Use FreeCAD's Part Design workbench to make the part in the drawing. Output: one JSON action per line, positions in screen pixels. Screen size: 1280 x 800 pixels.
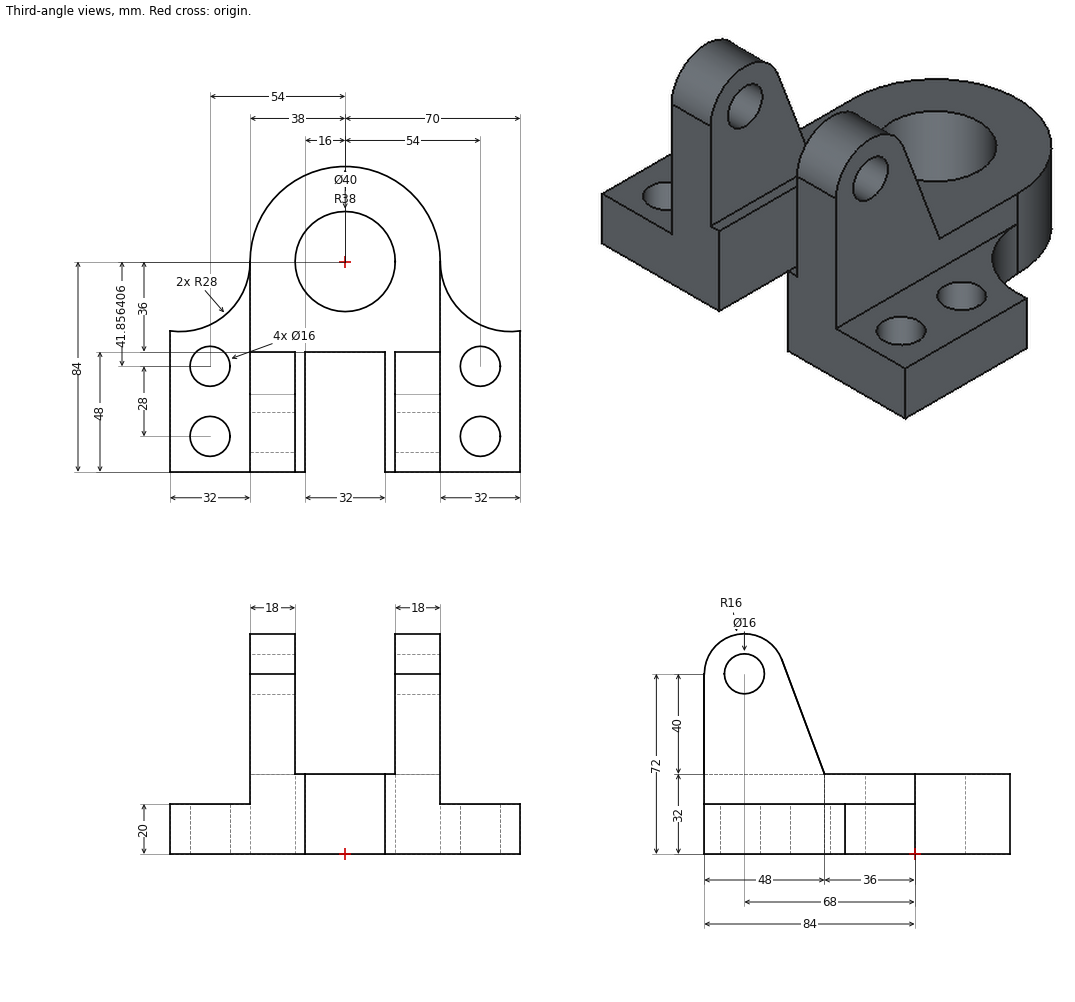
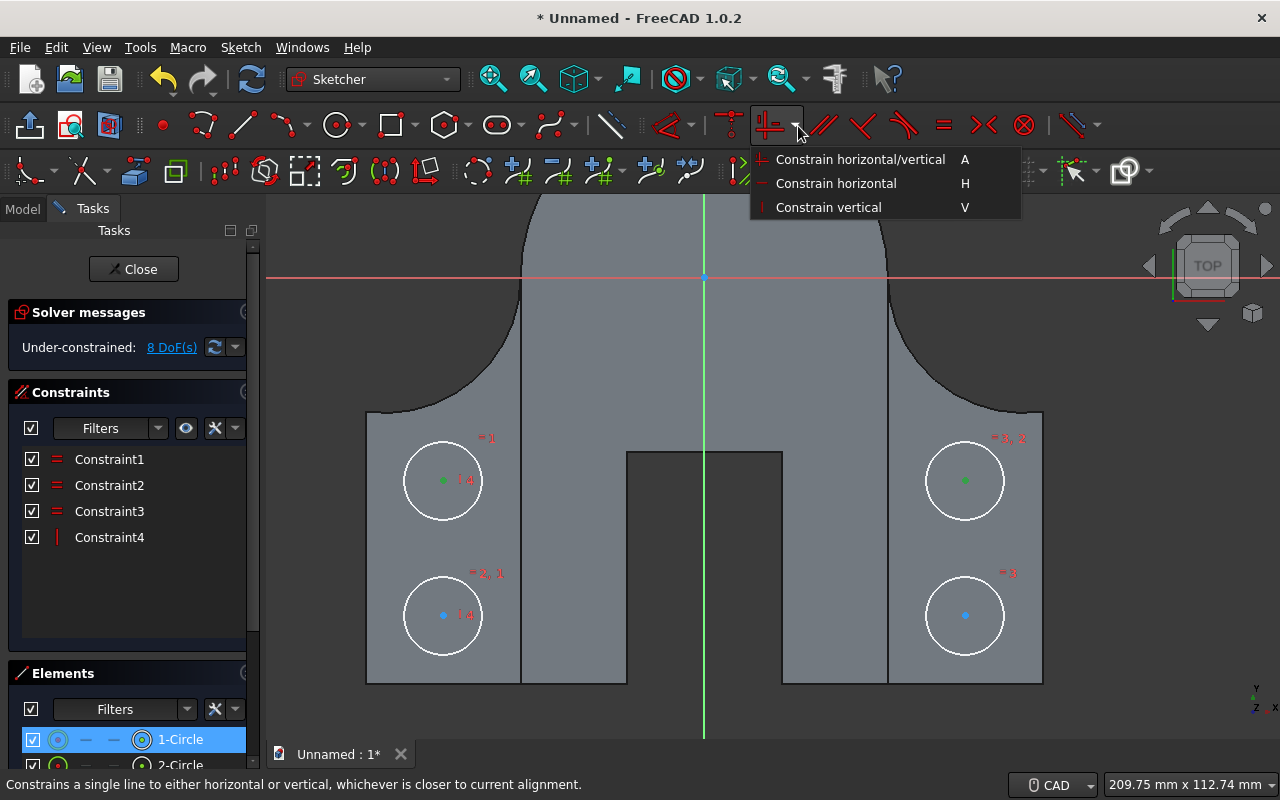
{"action": "left_click", "coordinate": [886, 183]}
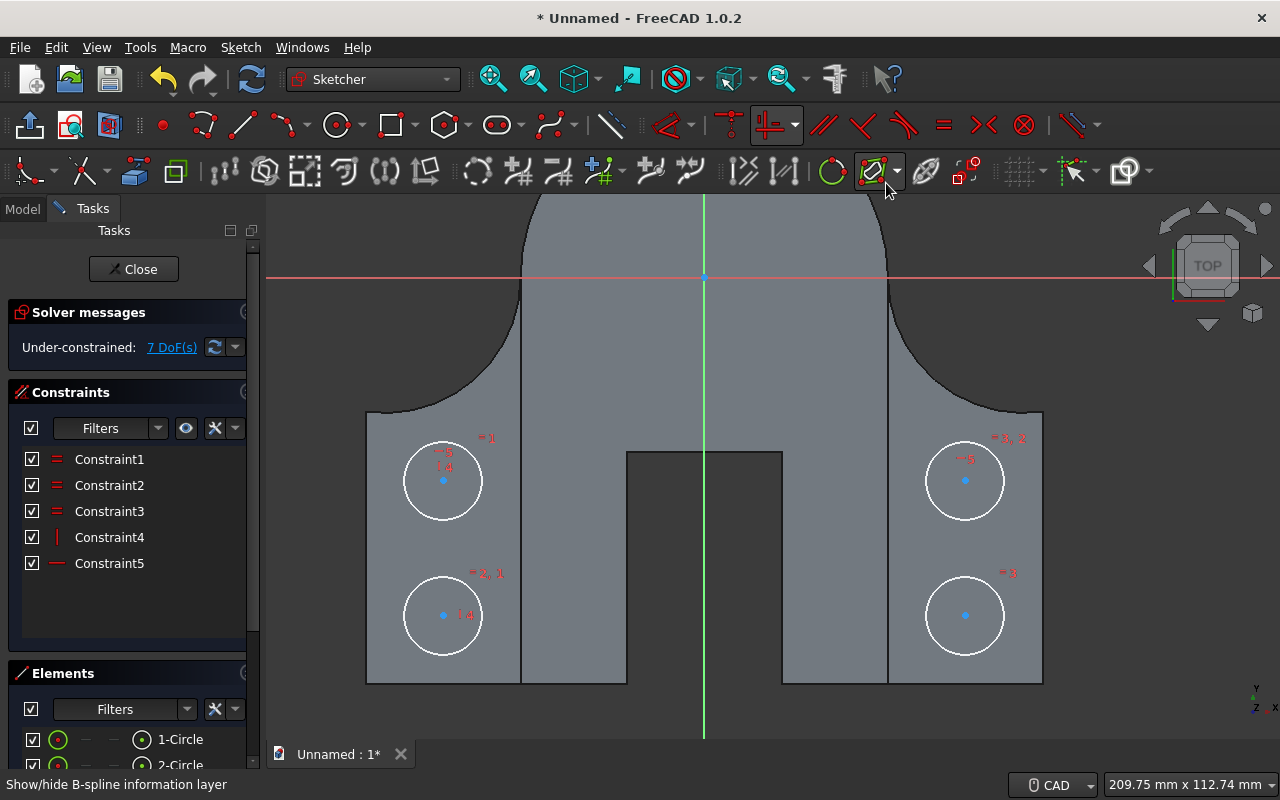
{"action": "left_click", "coordinate": [965, 481]}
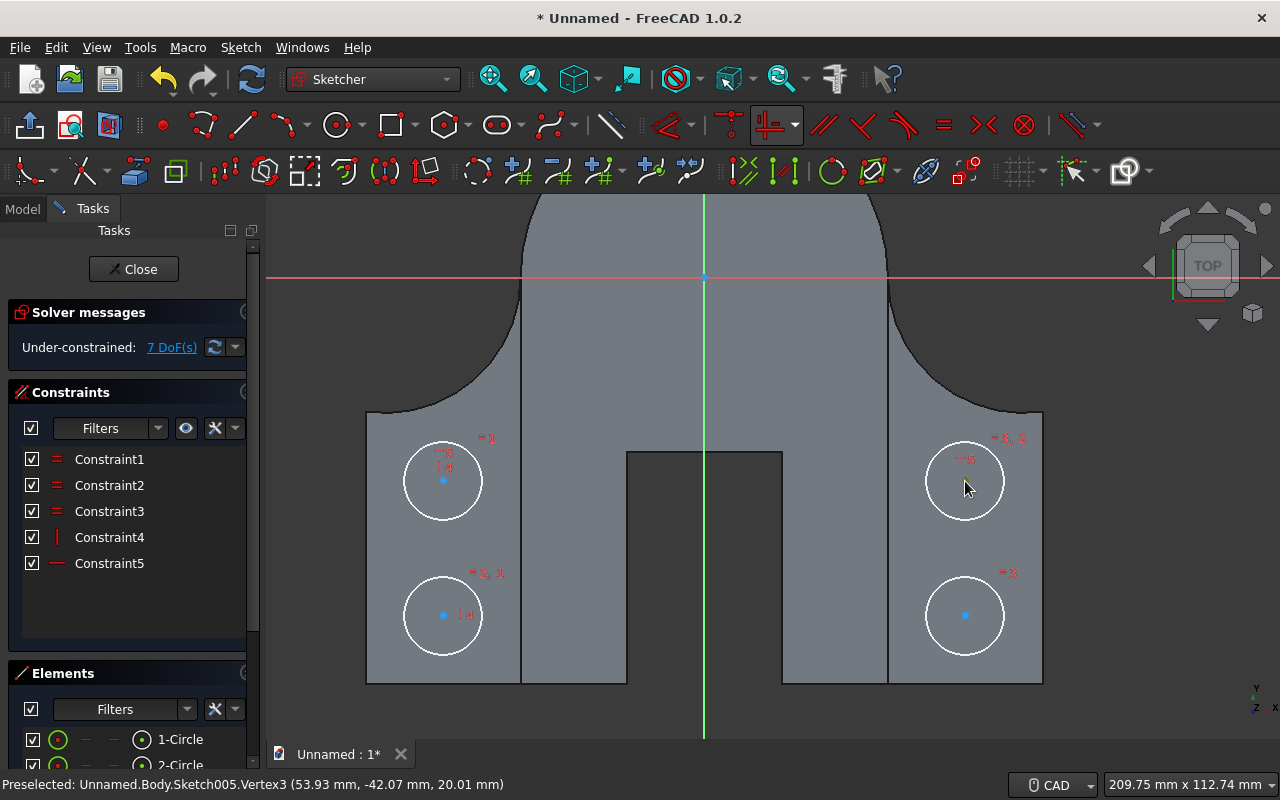
{"action": "left_click", "coordinate": [965, 616]}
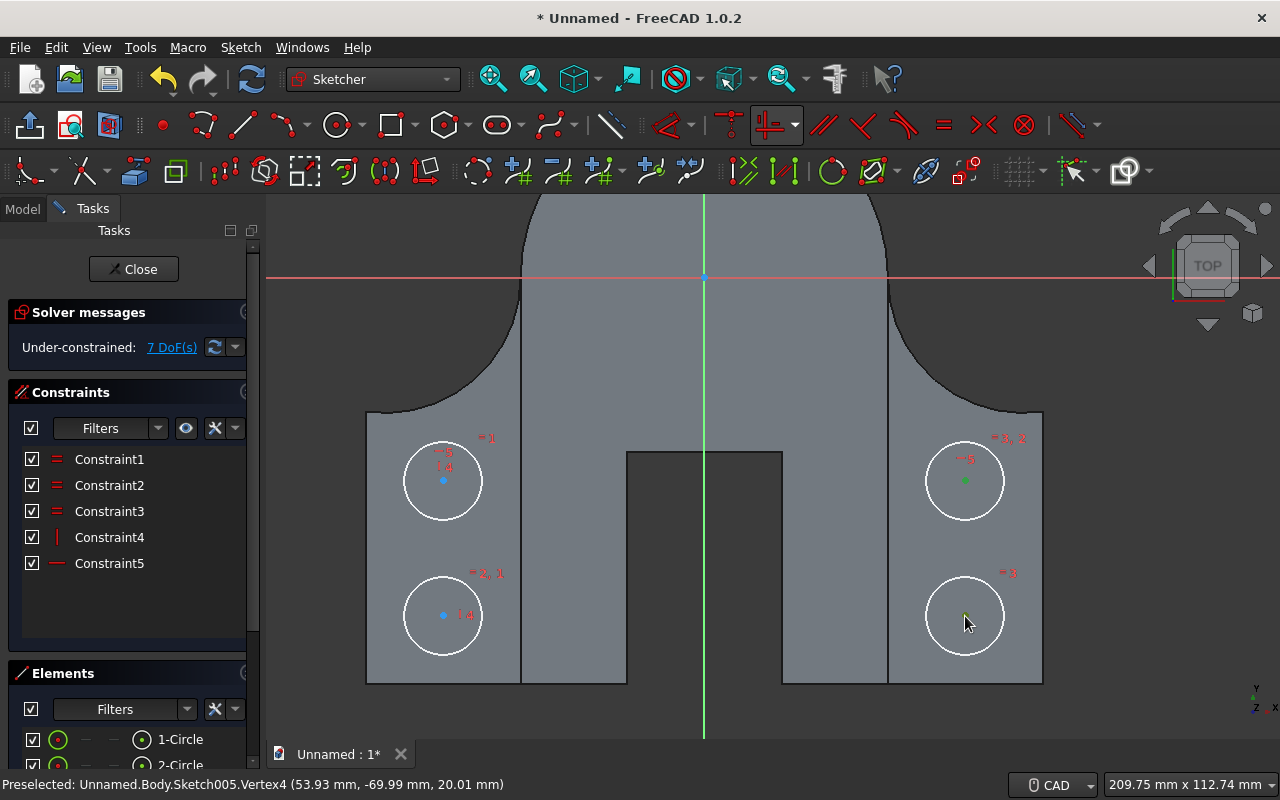
{"action": "left_click", "coordinate": [798, 126]}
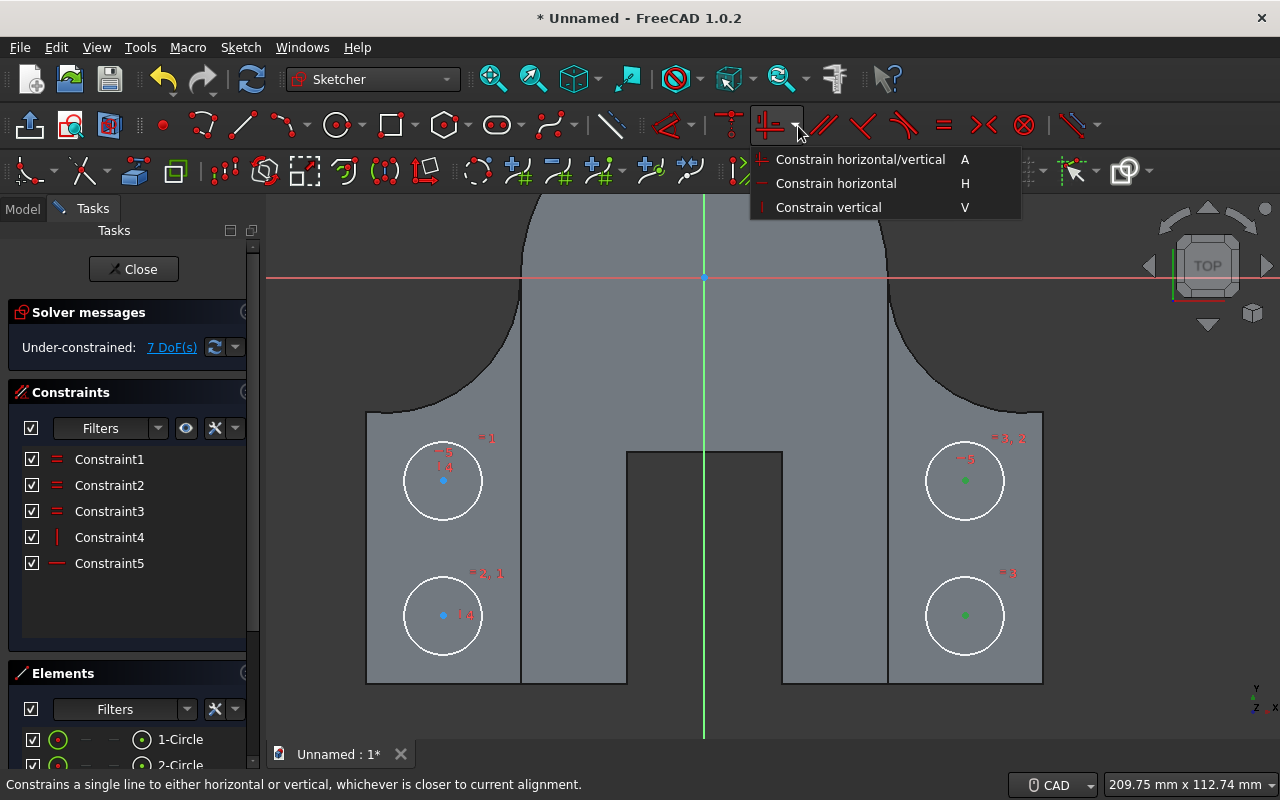
{"action": "left_click", "coordinate": [886, 207]}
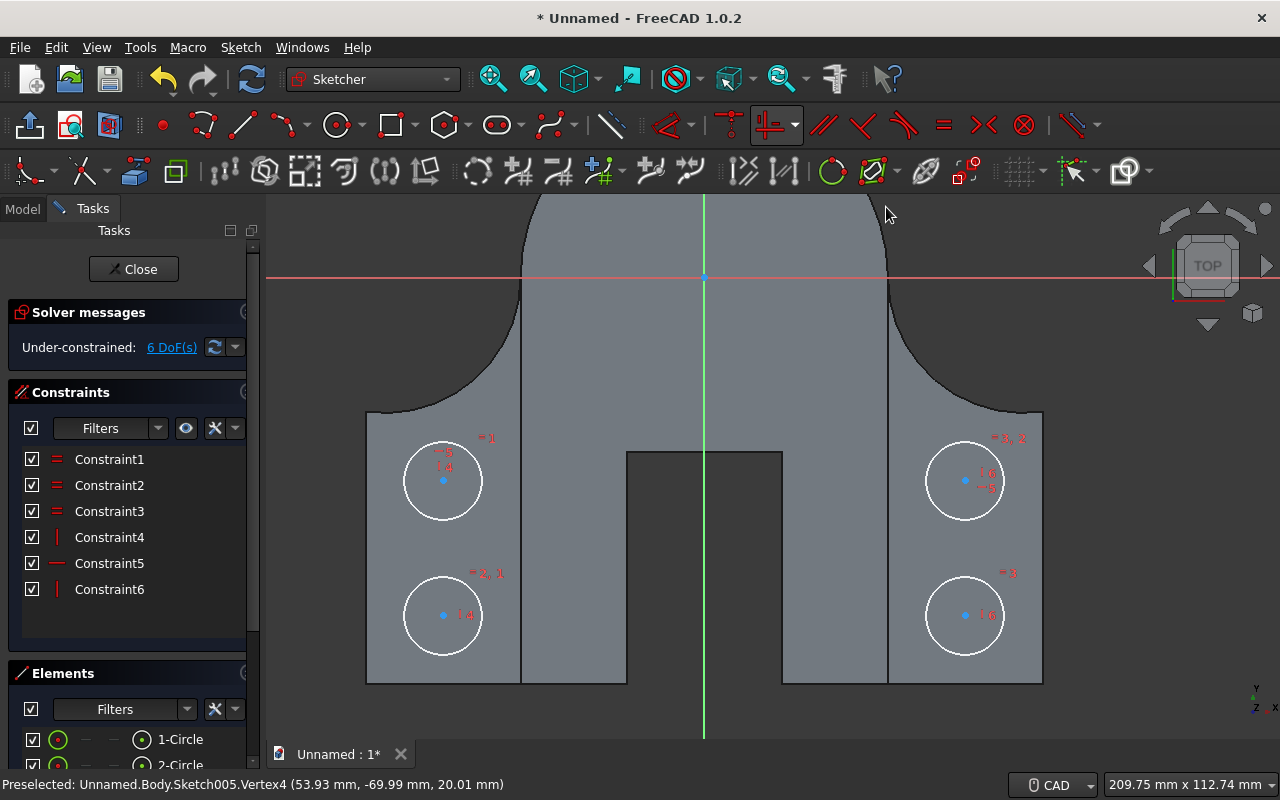
{"action": "left_click", "coordinate": [443, 616]}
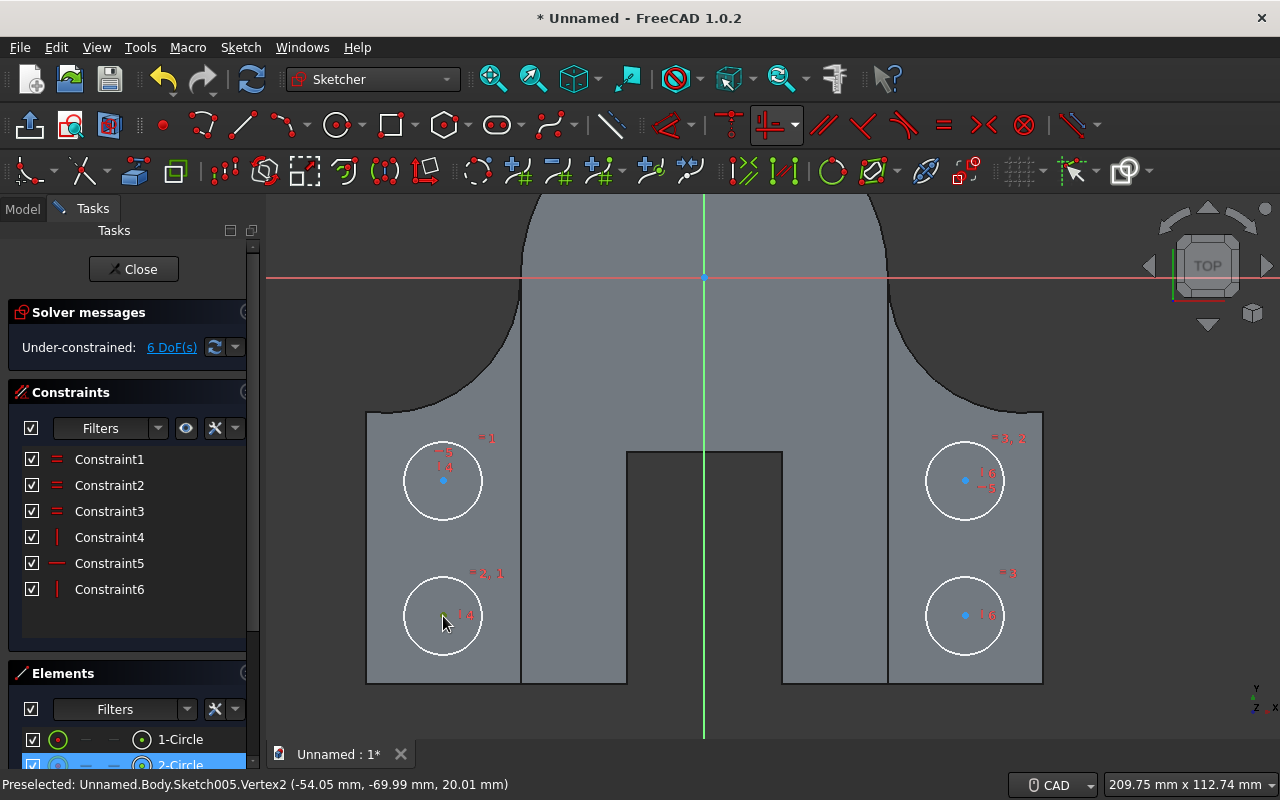
{"action": "left_click", "coordinate": [965, 616]}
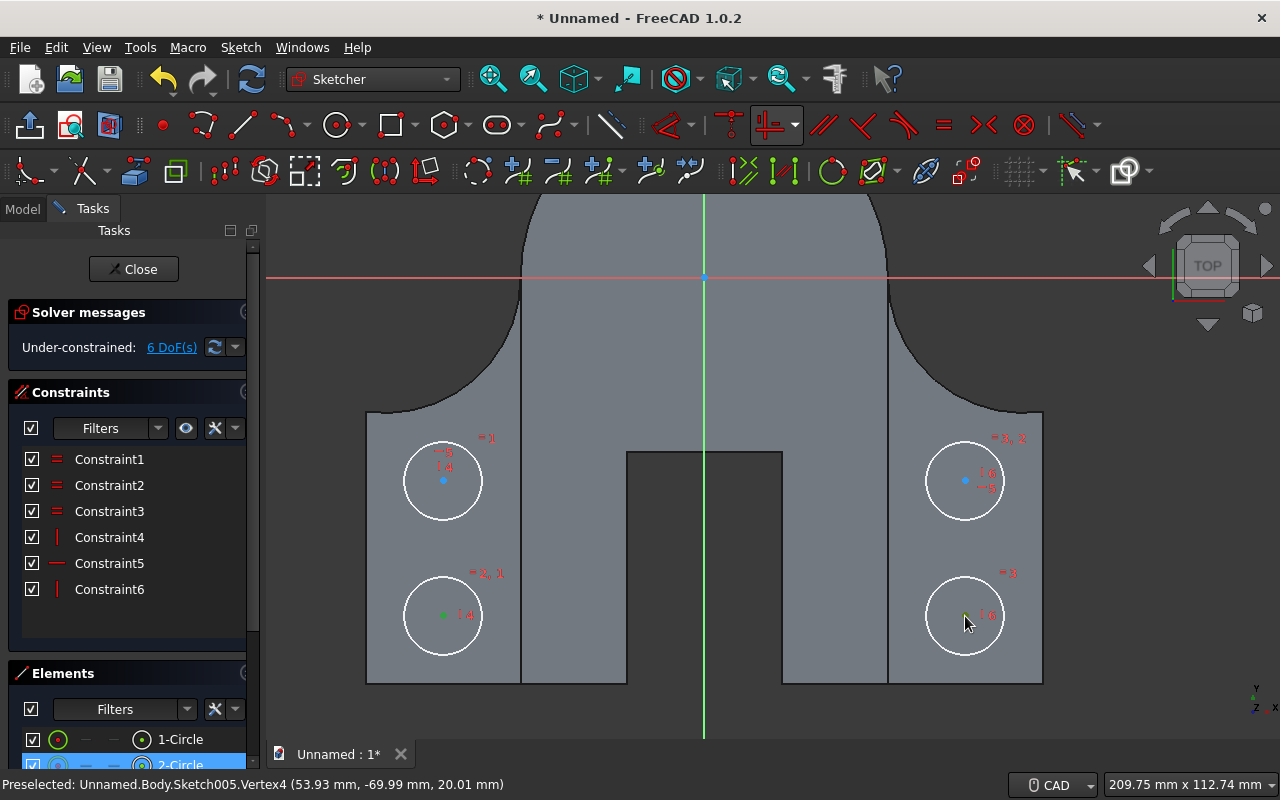
{"action": "key", "text": "h"}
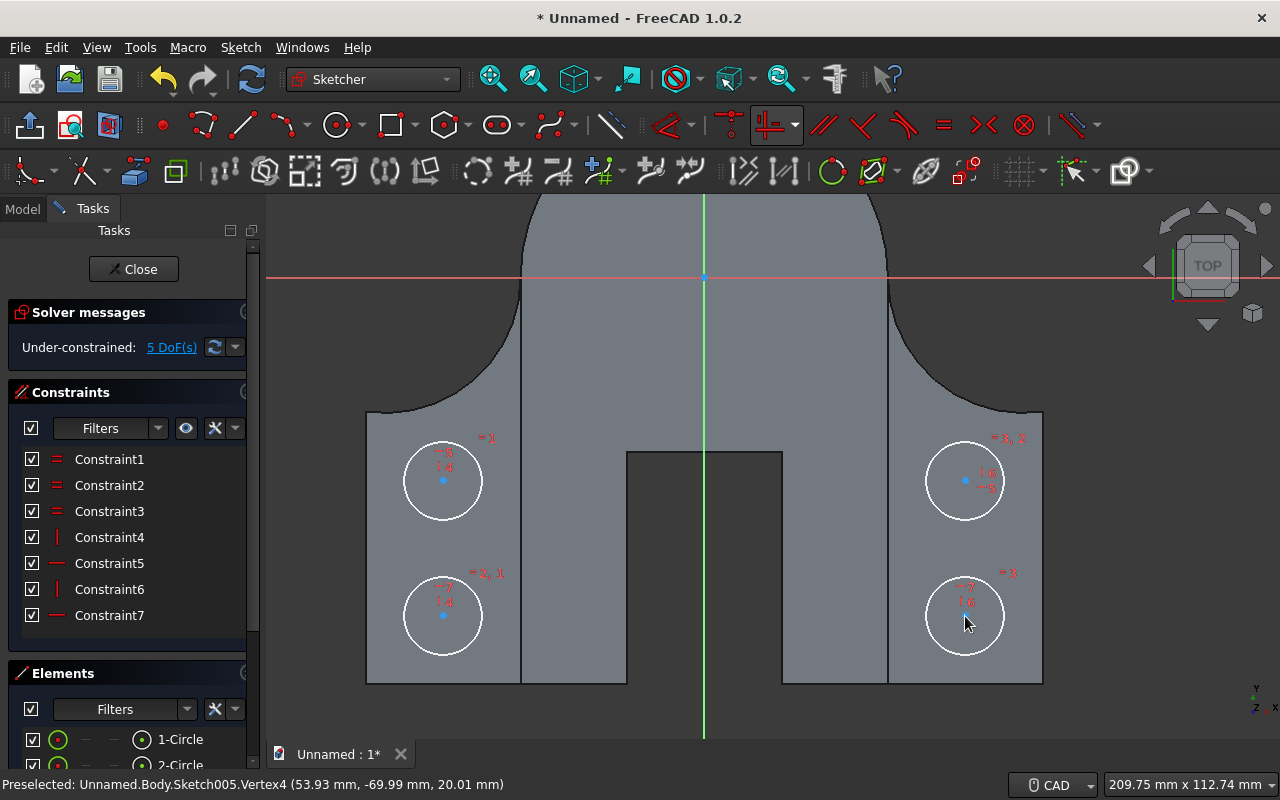
{"action": "left_click", "coordinate": [666, 126]}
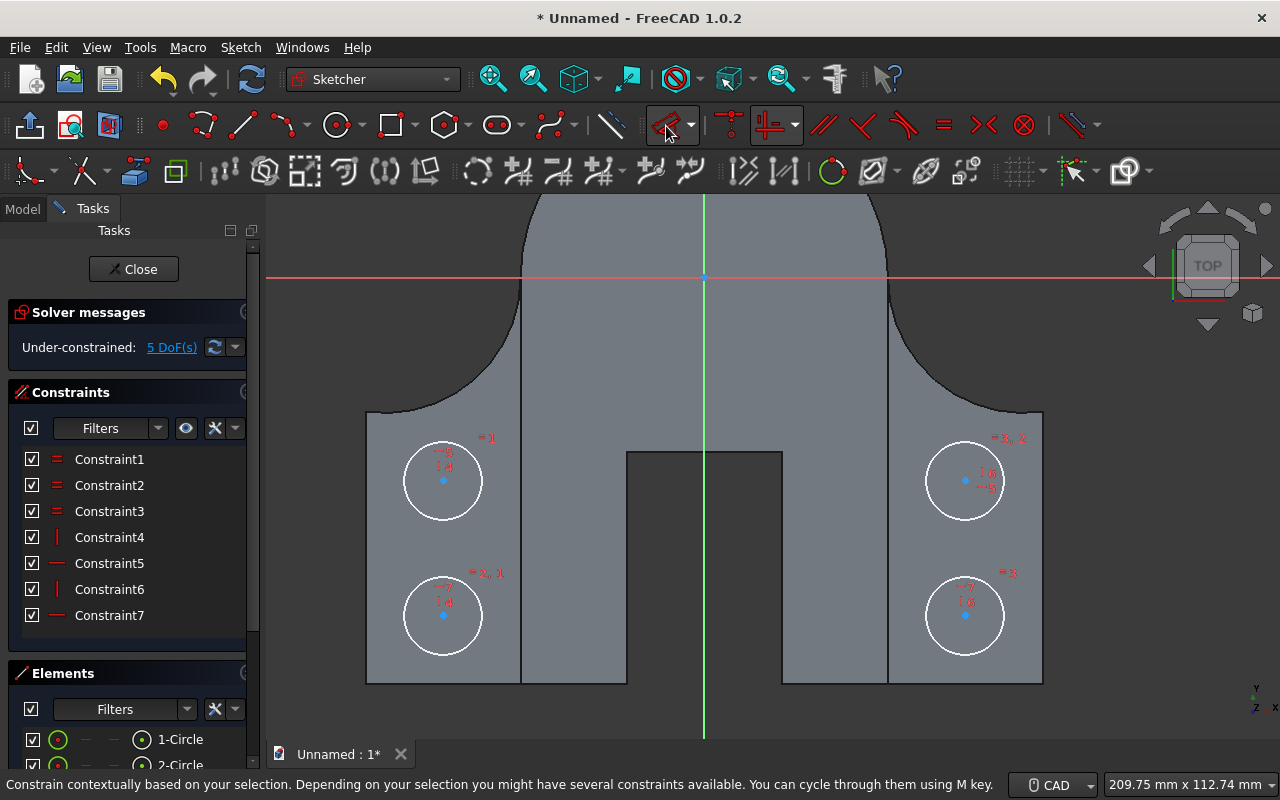
{"action": "left_click", "coordinate": [470, 453]}
{"action": "left_click", "coordinate": [492, 430]}